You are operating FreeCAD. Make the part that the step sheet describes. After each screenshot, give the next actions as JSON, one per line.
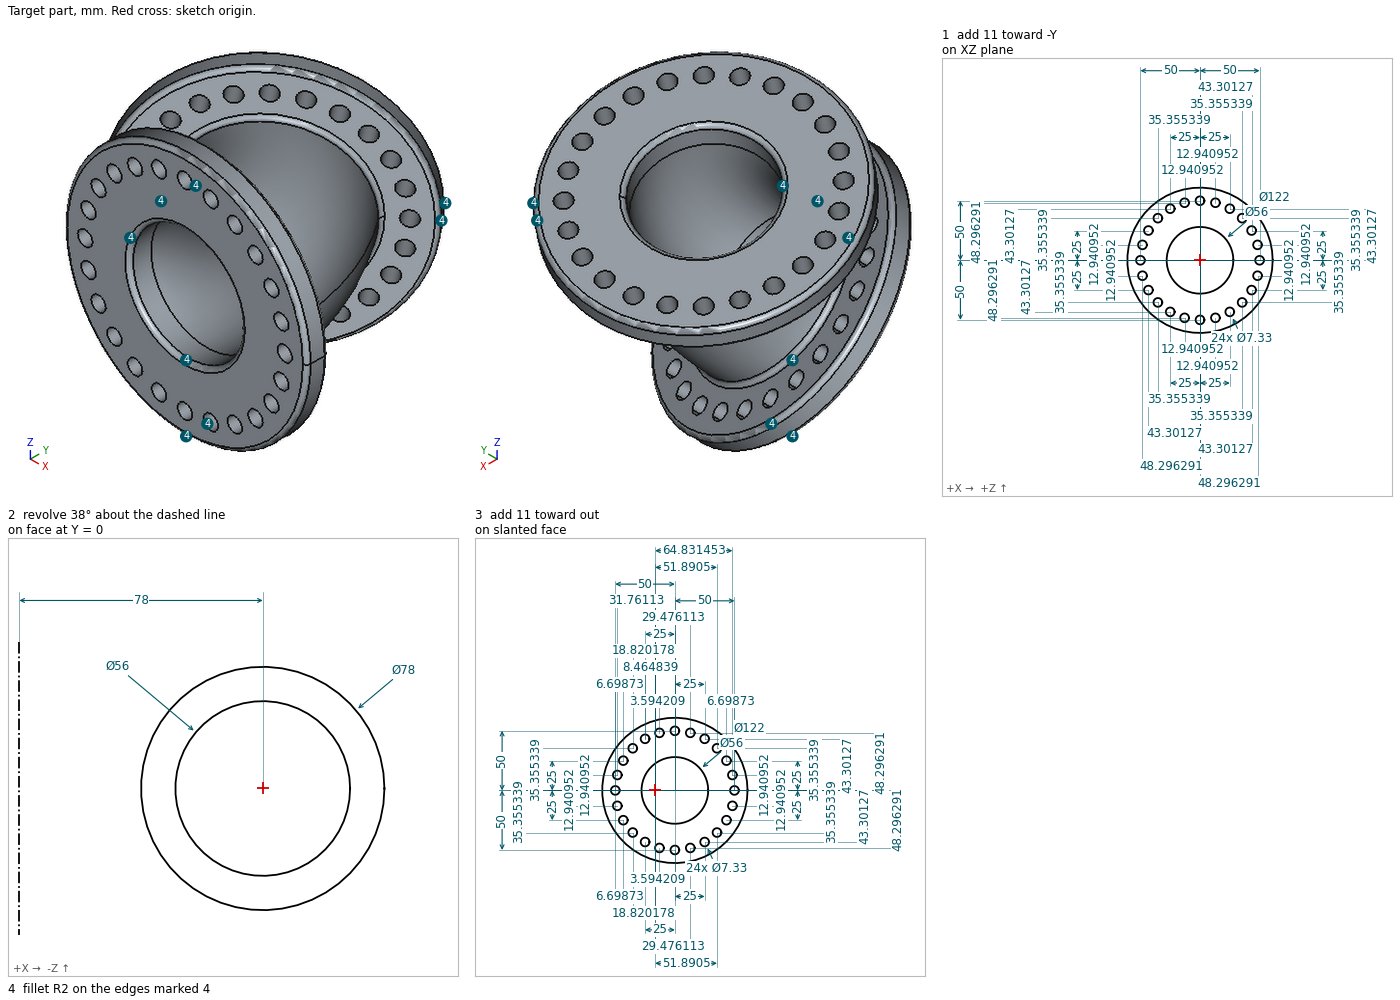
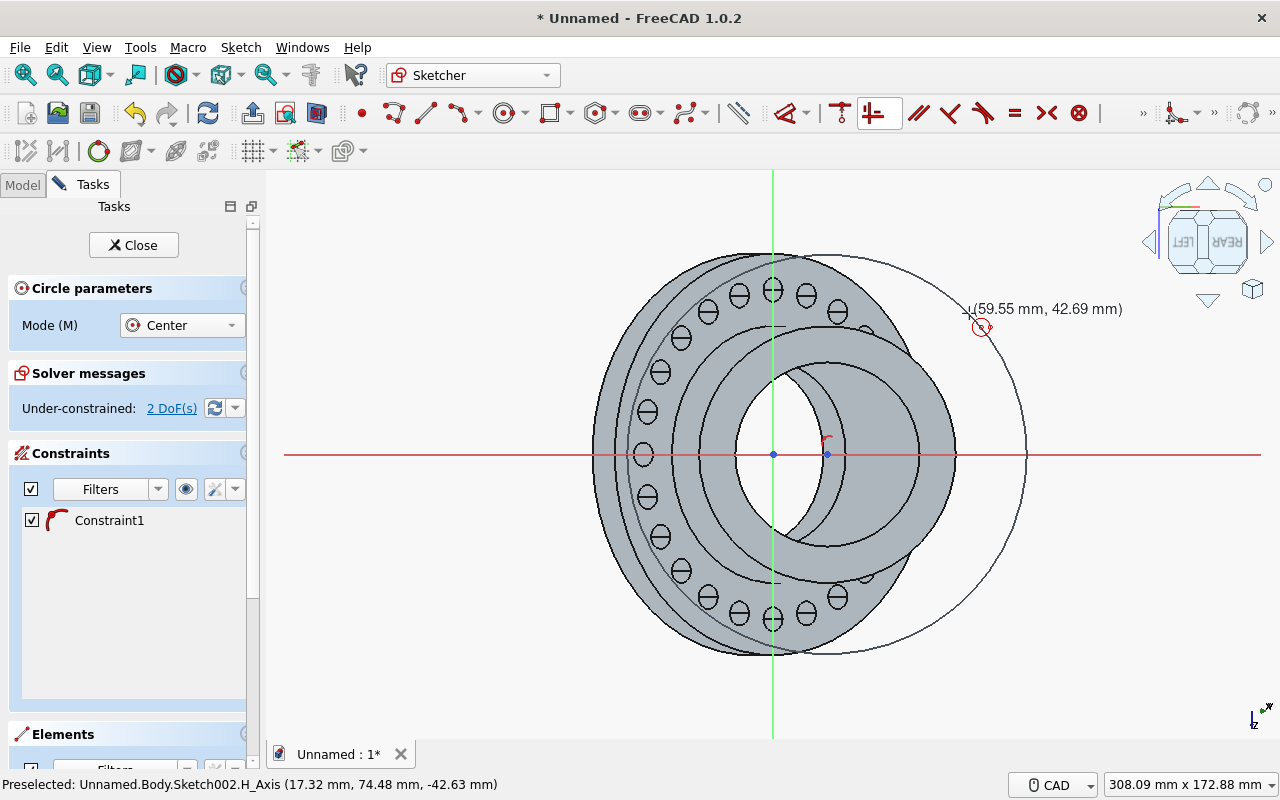
{"action": "scroll", "coordinate": [944, 338], "scroll_direction": "up", "scroll_amount": 4}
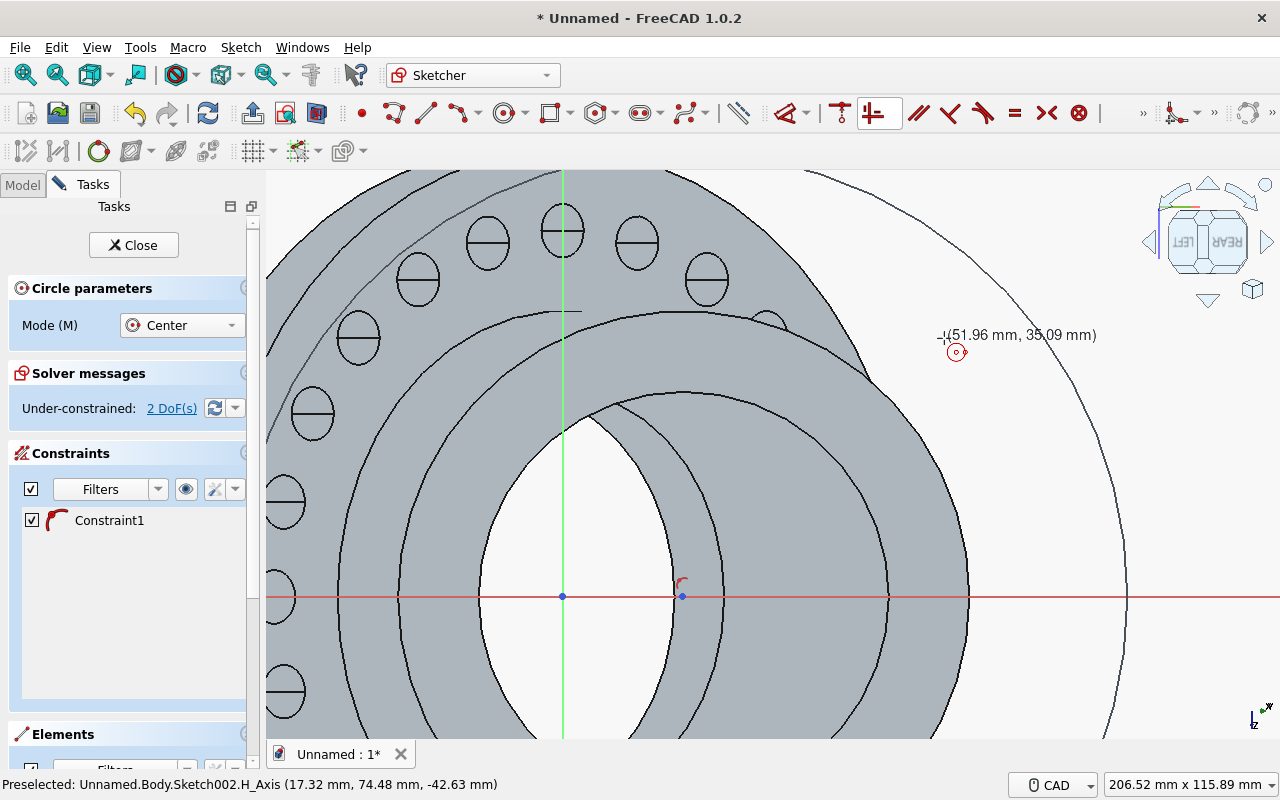
{"action": "left_click", "coordinate": [943, 338]}
{"action": "left_click", "coordinate": [962, 319]}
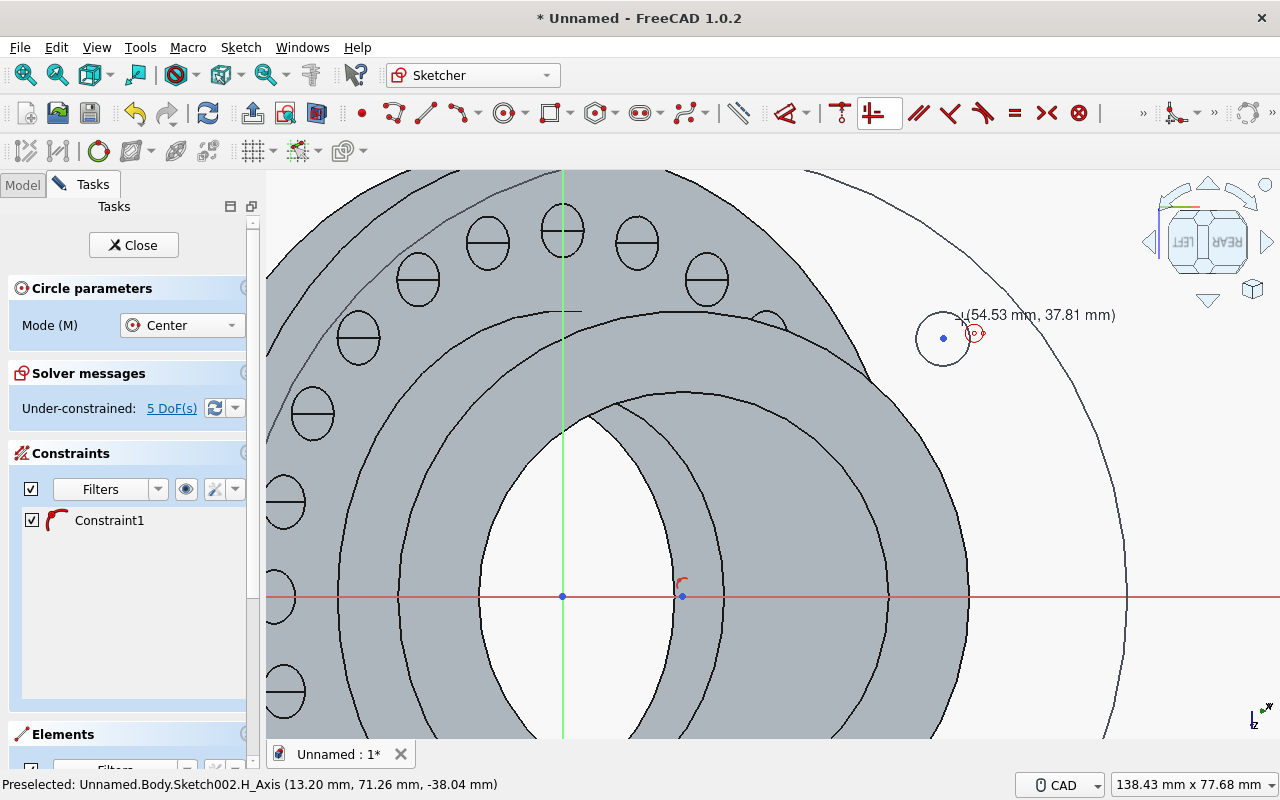
{"action": "left_click", "coordinate": [867, 280]}
{"action": "left_click", "coordinate": [886, 261]}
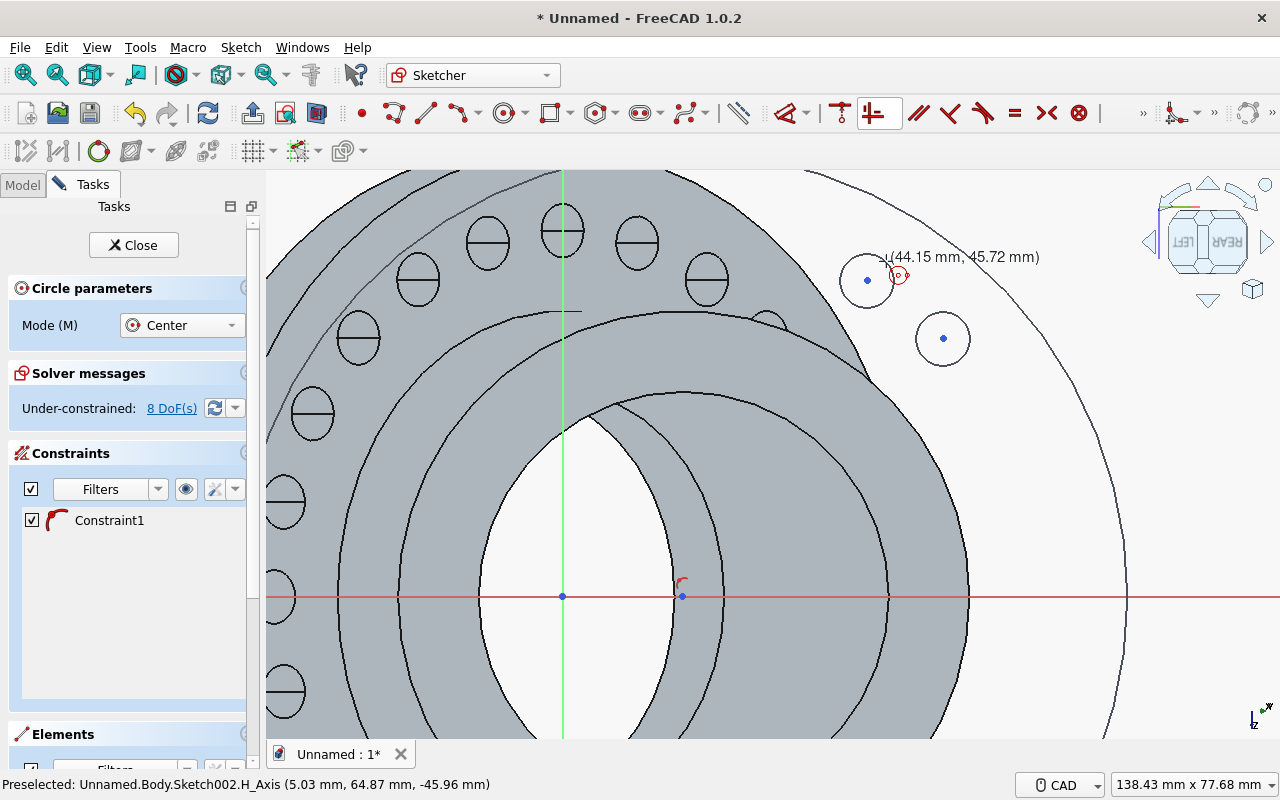
{"action": "left_click", "coordinate": [779, 243]}
{"action": "left_click", "coordinate": [797, 224]}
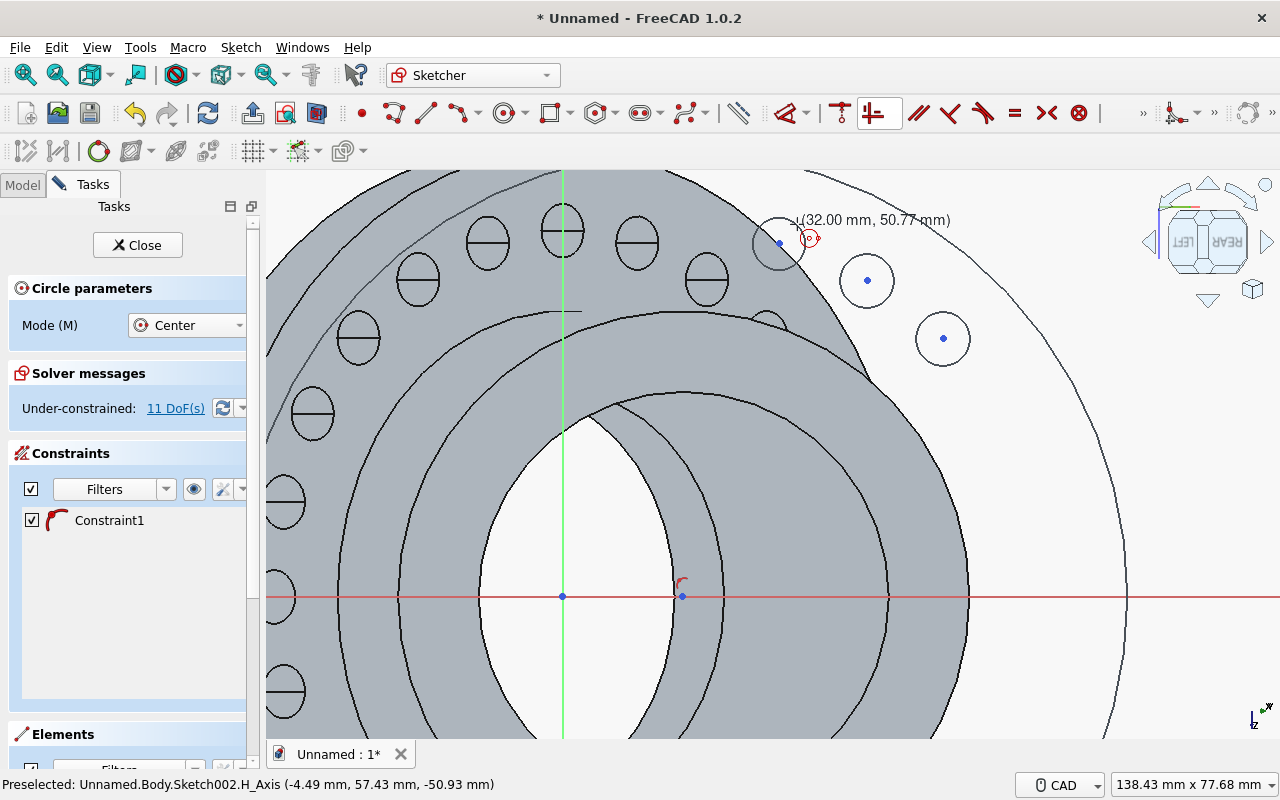
{"action": "left_click", "coordinate": [1001, 414]}
{"action": "left_click", "coordinate": [1020, 395]}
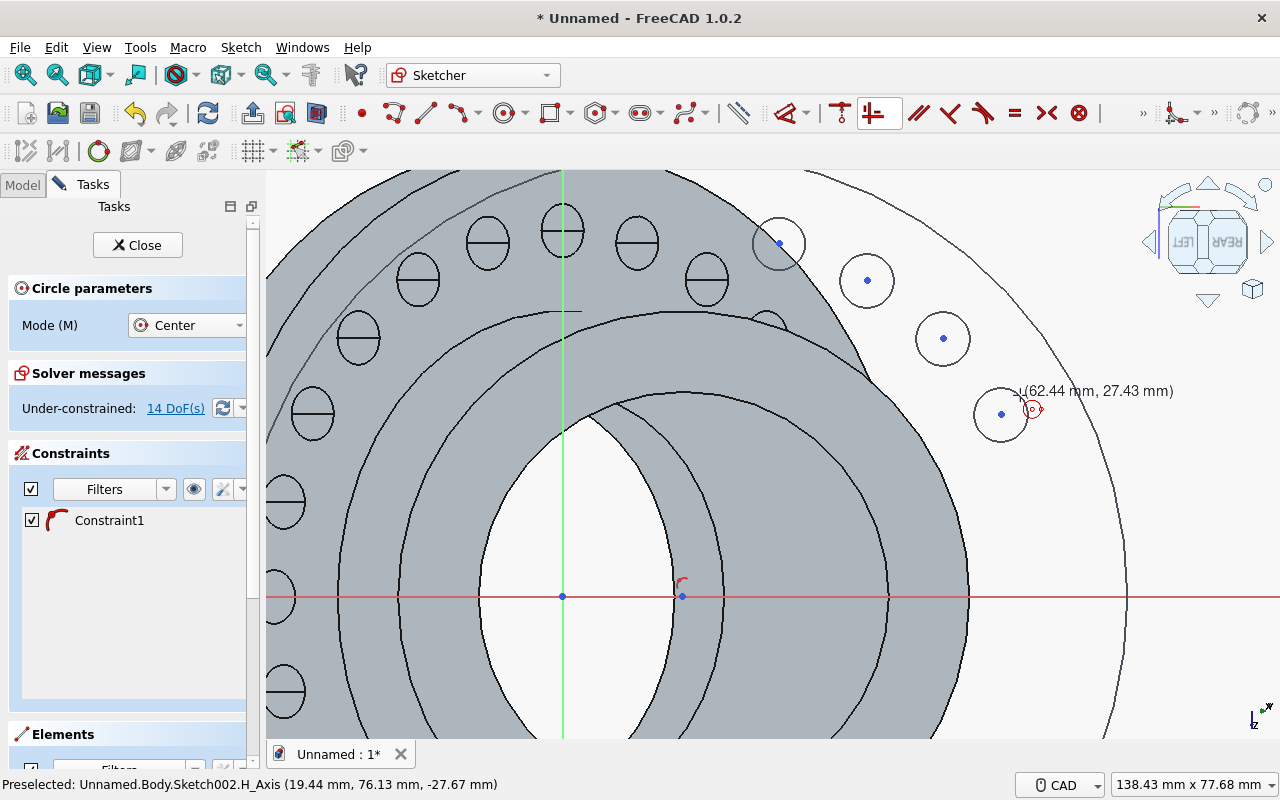
{"action": "left_click", "coordinate": [1037, 502]}
{"action": "left_click", "coordinate": [1056, 483]}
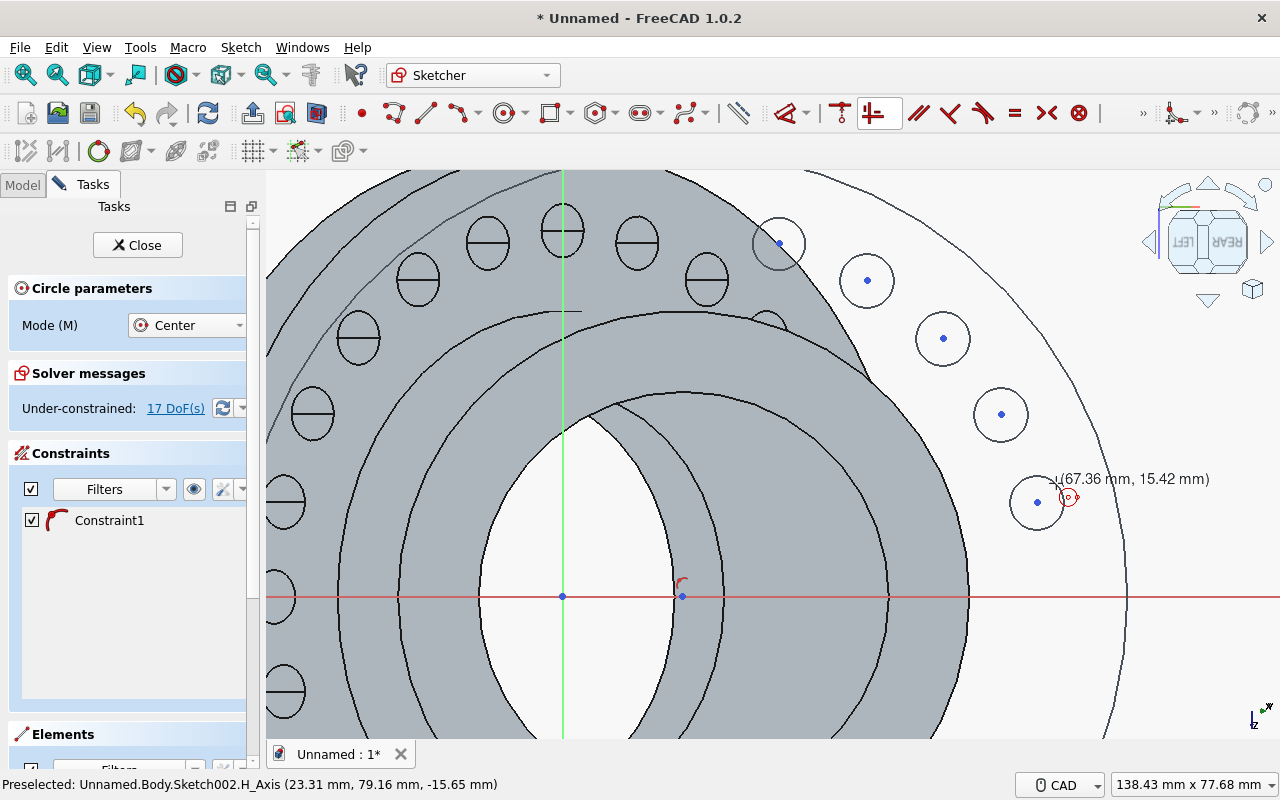
{"action": "left_click", "coordinate": [1050, 597]}
{"action": "left_click", "coordinate": [1069, 578]}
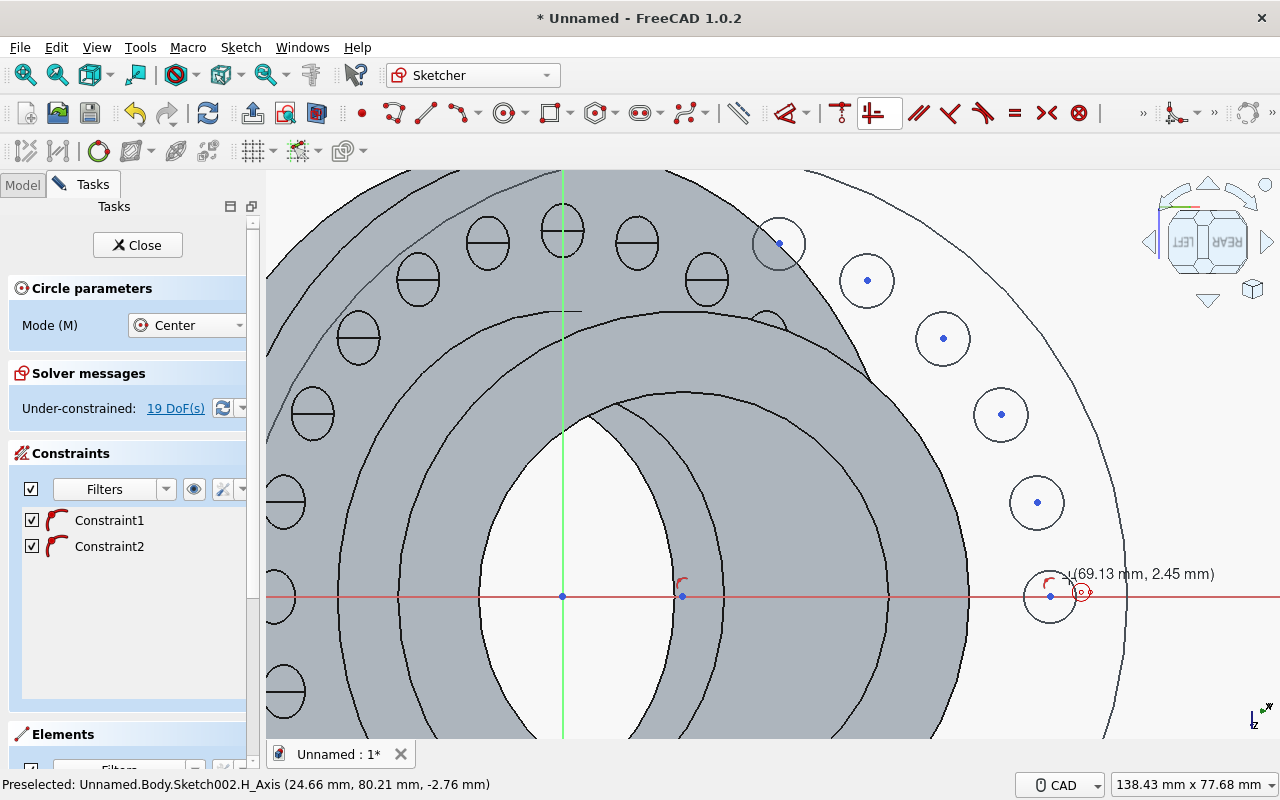
{"action": "left_click", "coordinate": [683, 597]}
{"action": "left_click", "coordinate": [829, 452]}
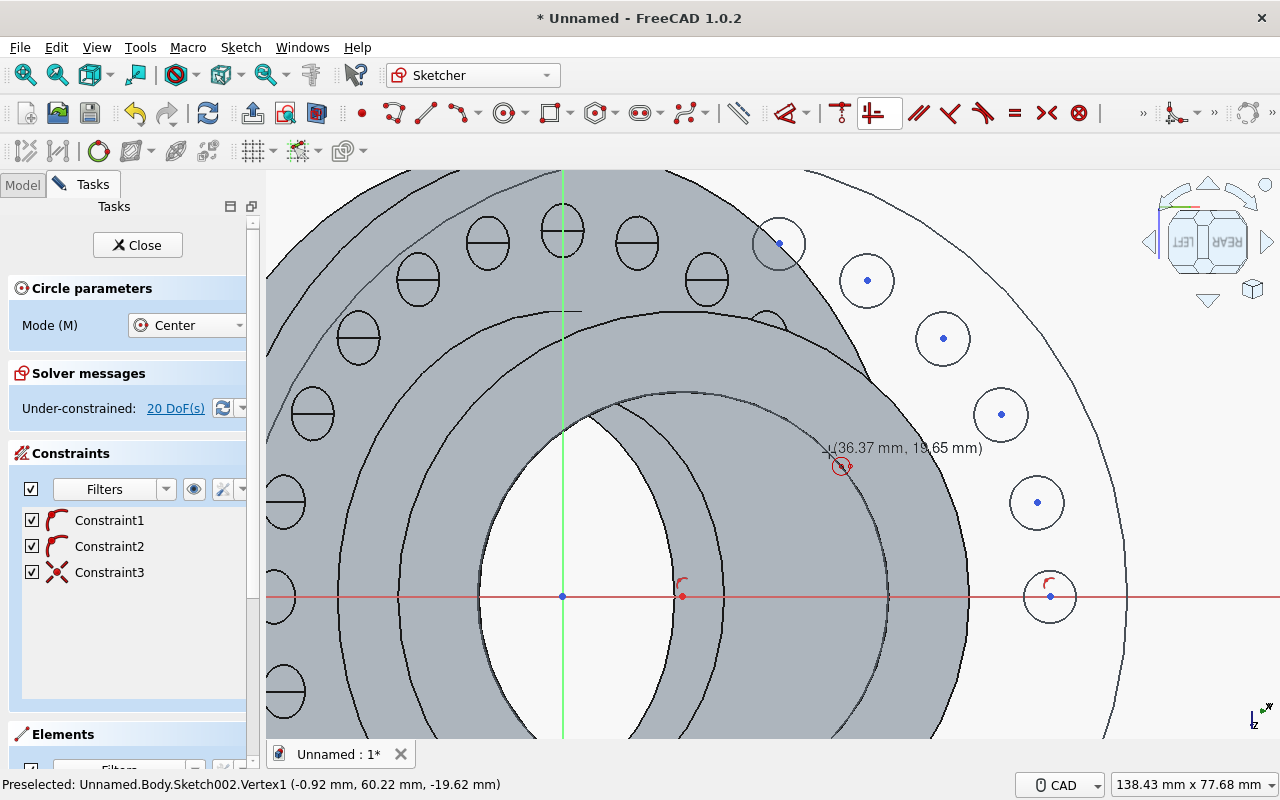
{"action": "left_click", "coordinate": [684, 231]}
{"action": "left_click", "coordinate": [703, 212]}